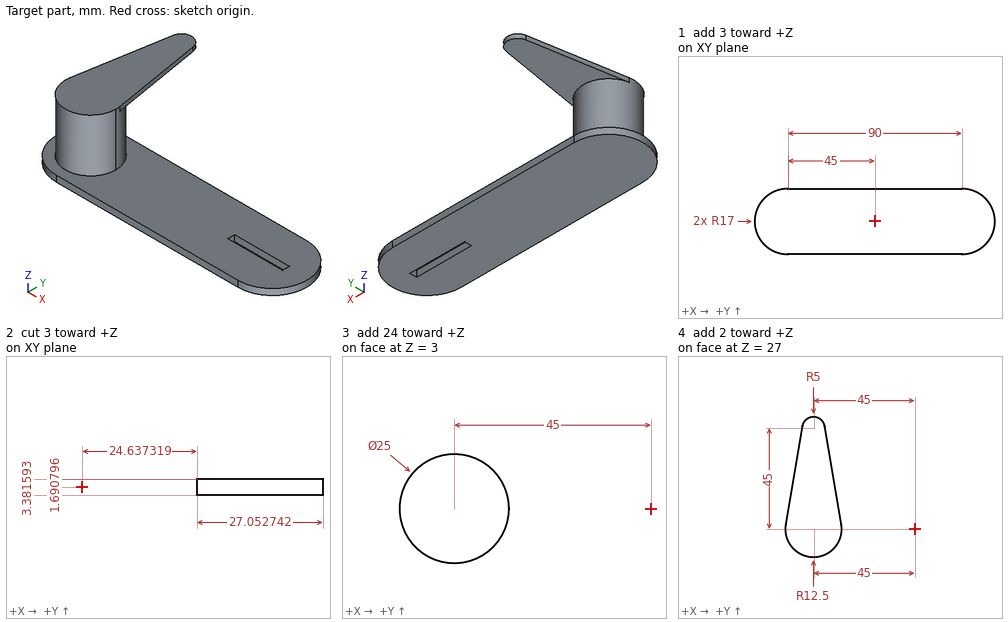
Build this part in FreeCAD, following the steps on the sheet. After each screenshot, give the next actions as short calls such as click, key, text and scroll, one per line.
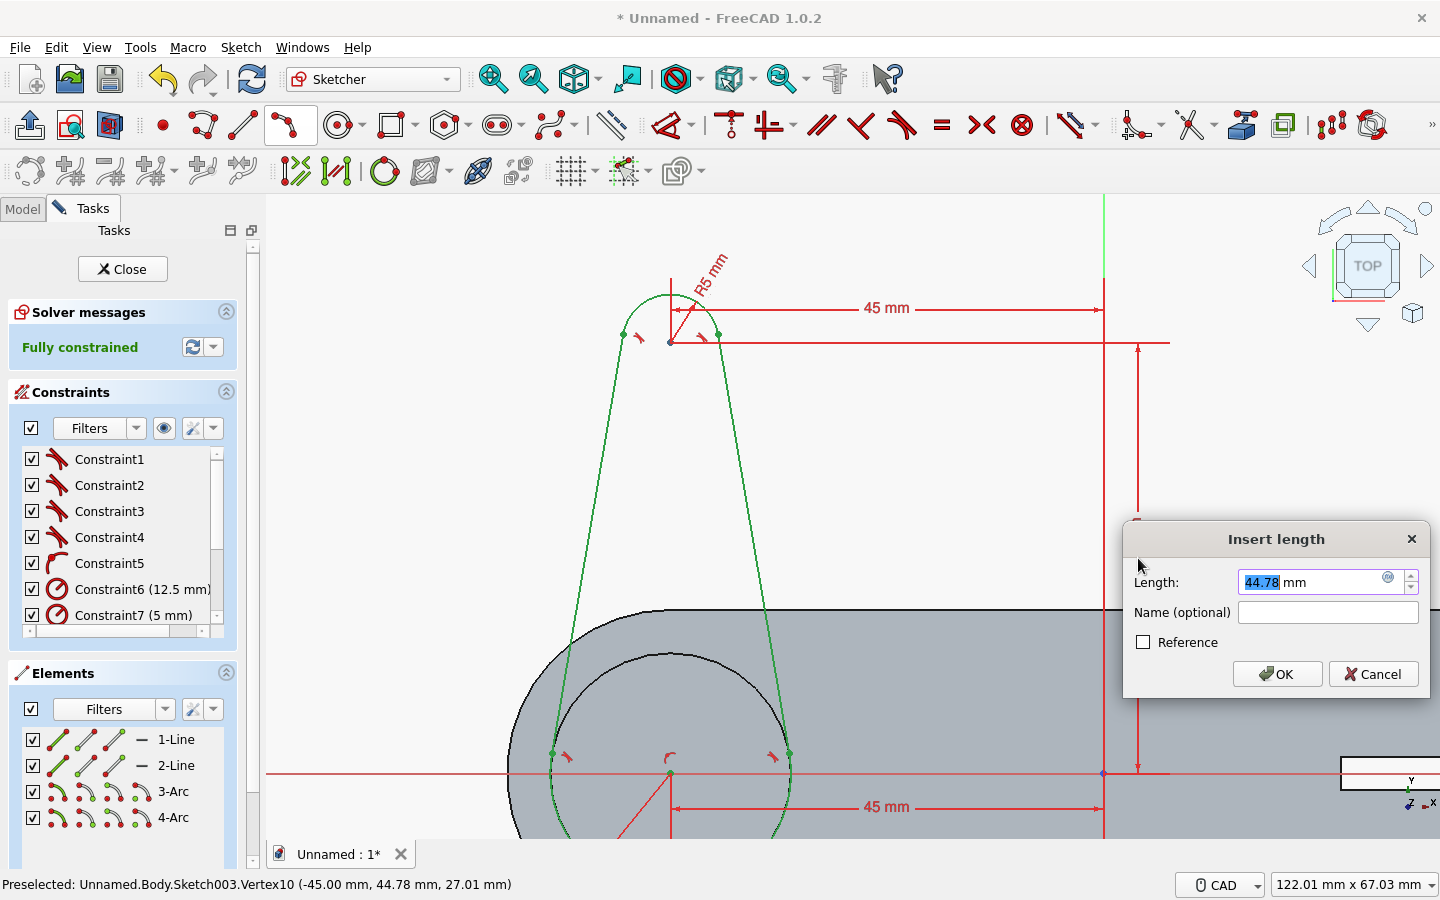
text(45)
key(Return)
key(Escape)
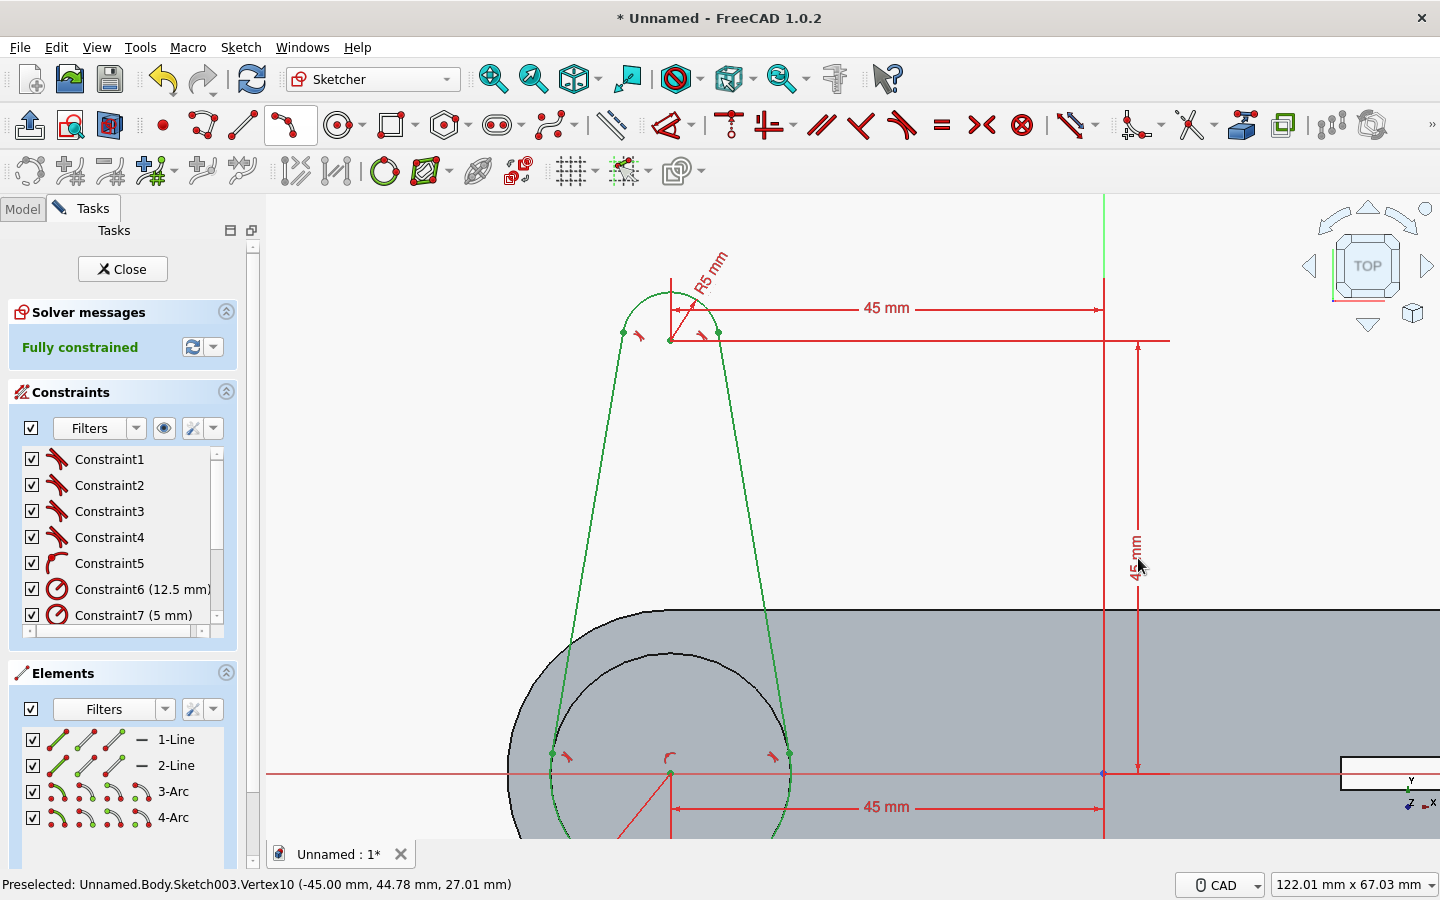
click(123, 269)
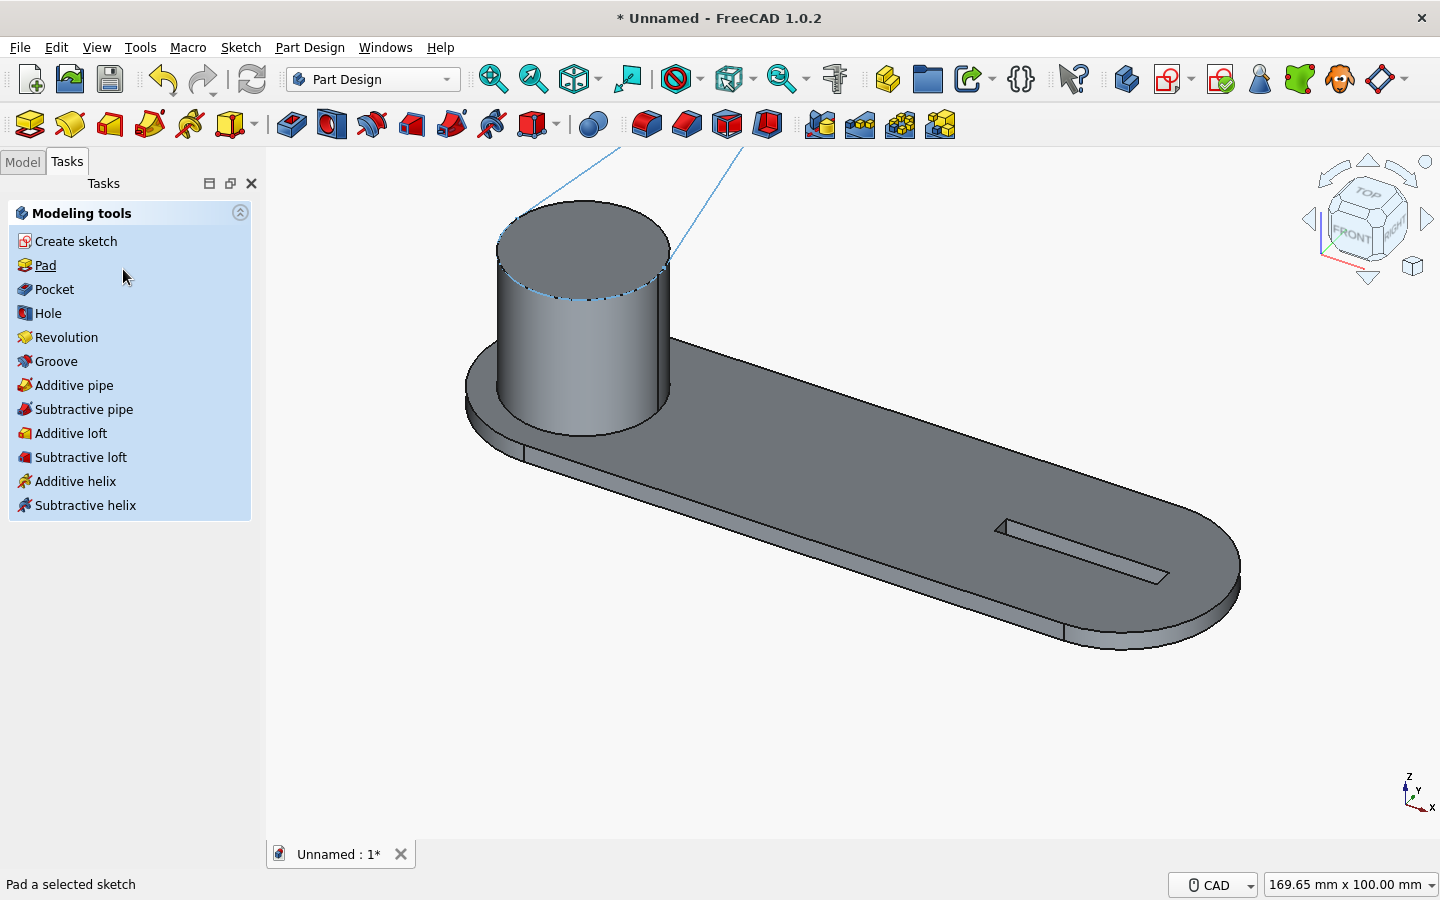
click(30, 124)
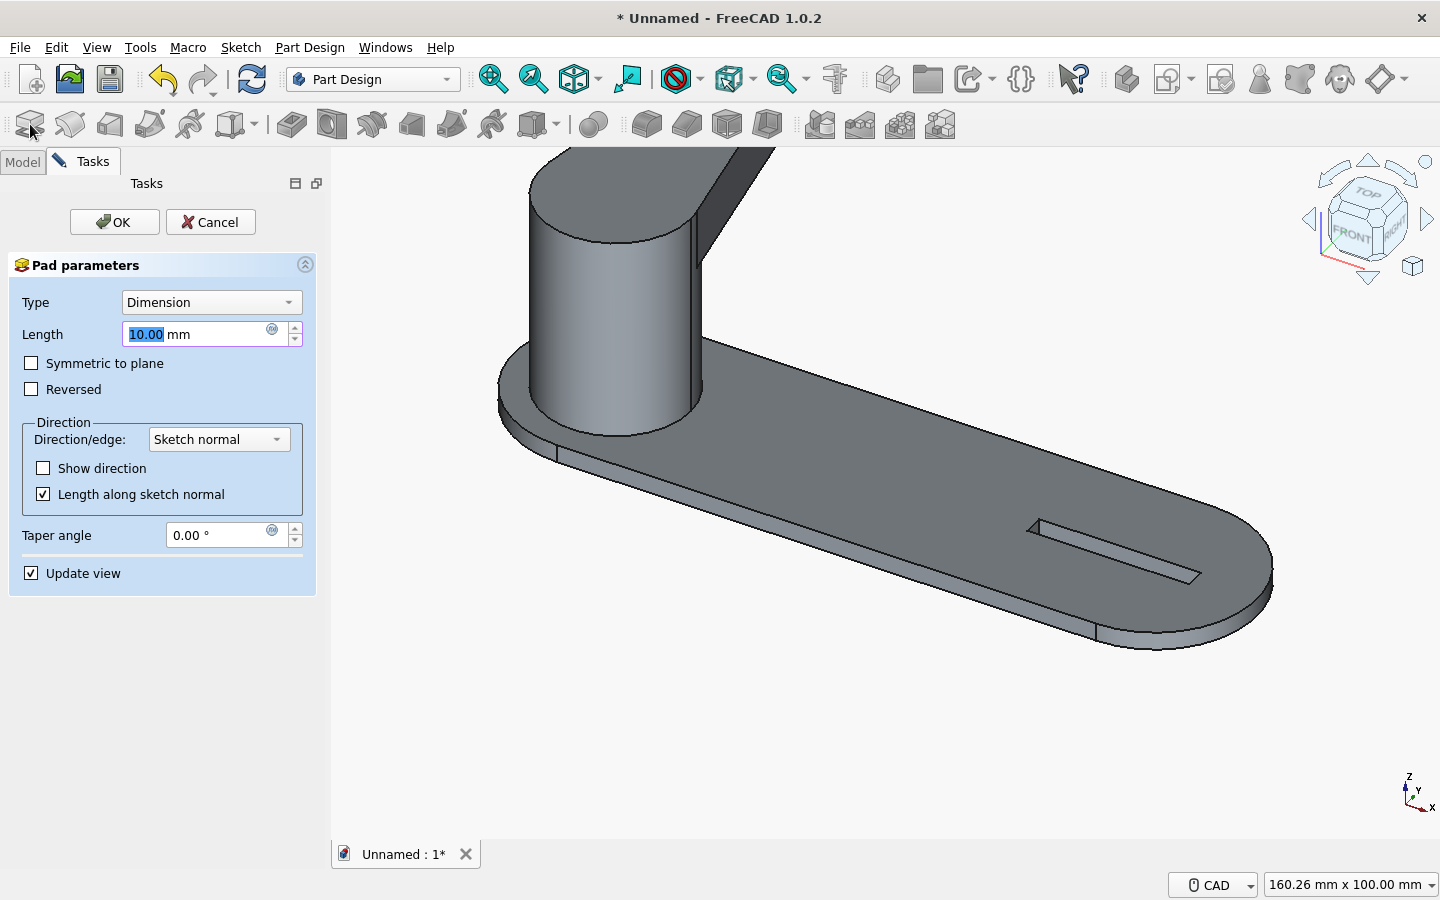
text(2)
key(Tab)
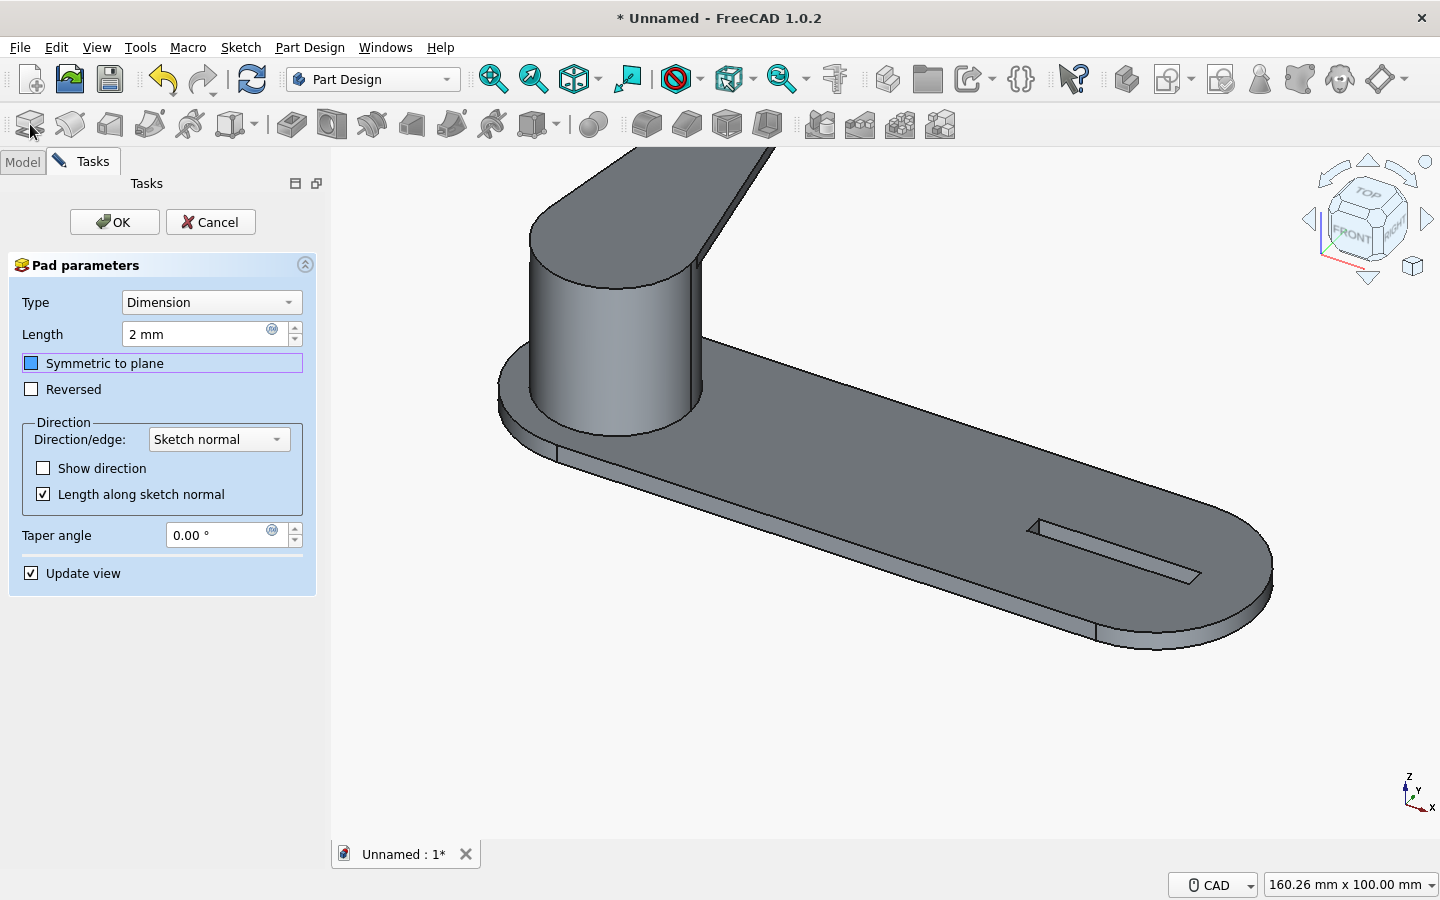
click(115, 222)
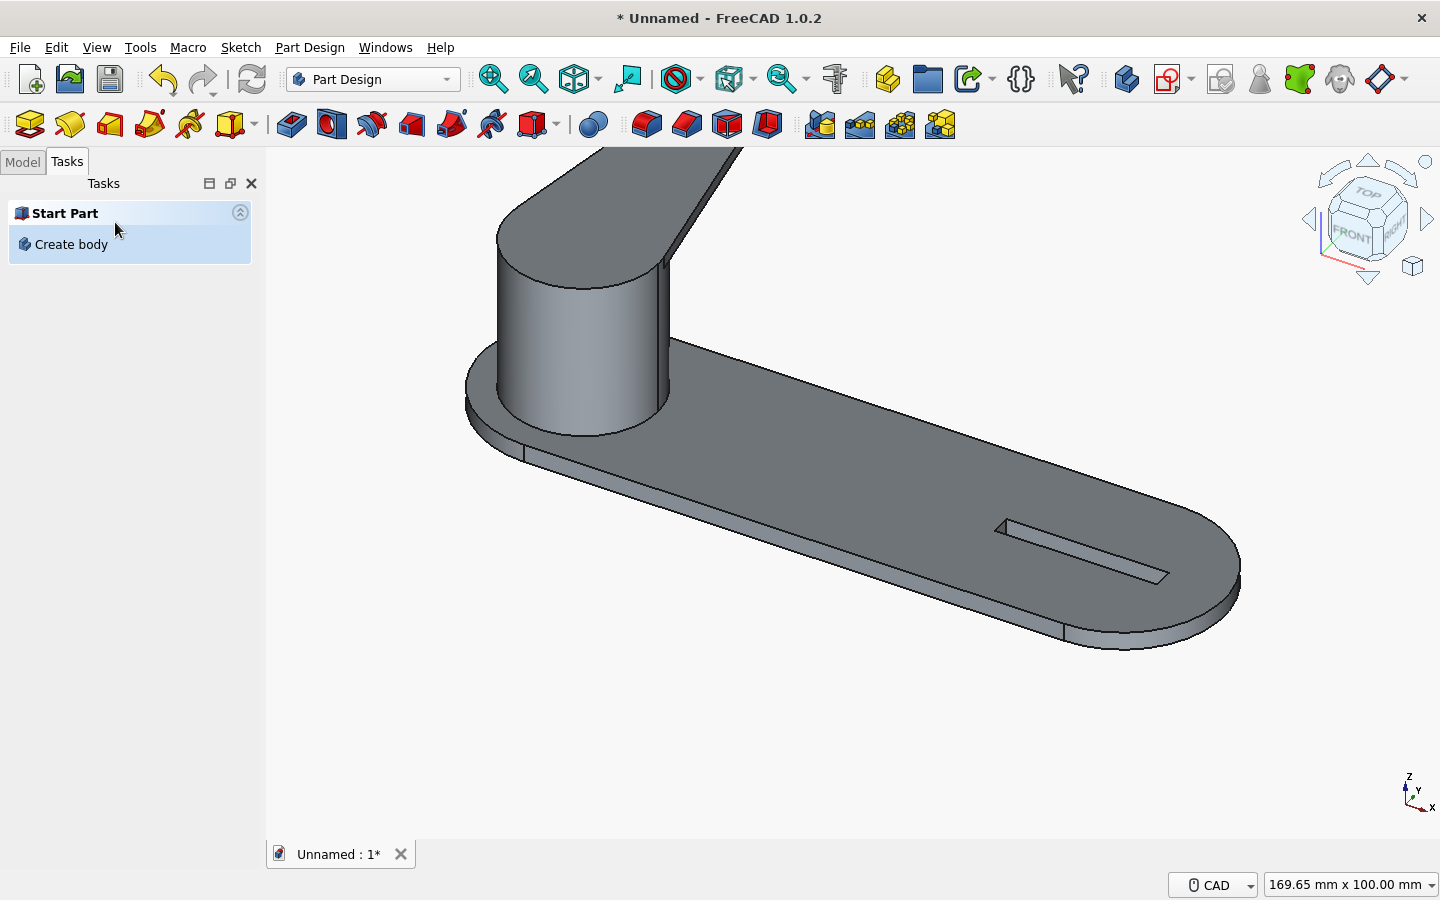
key(0)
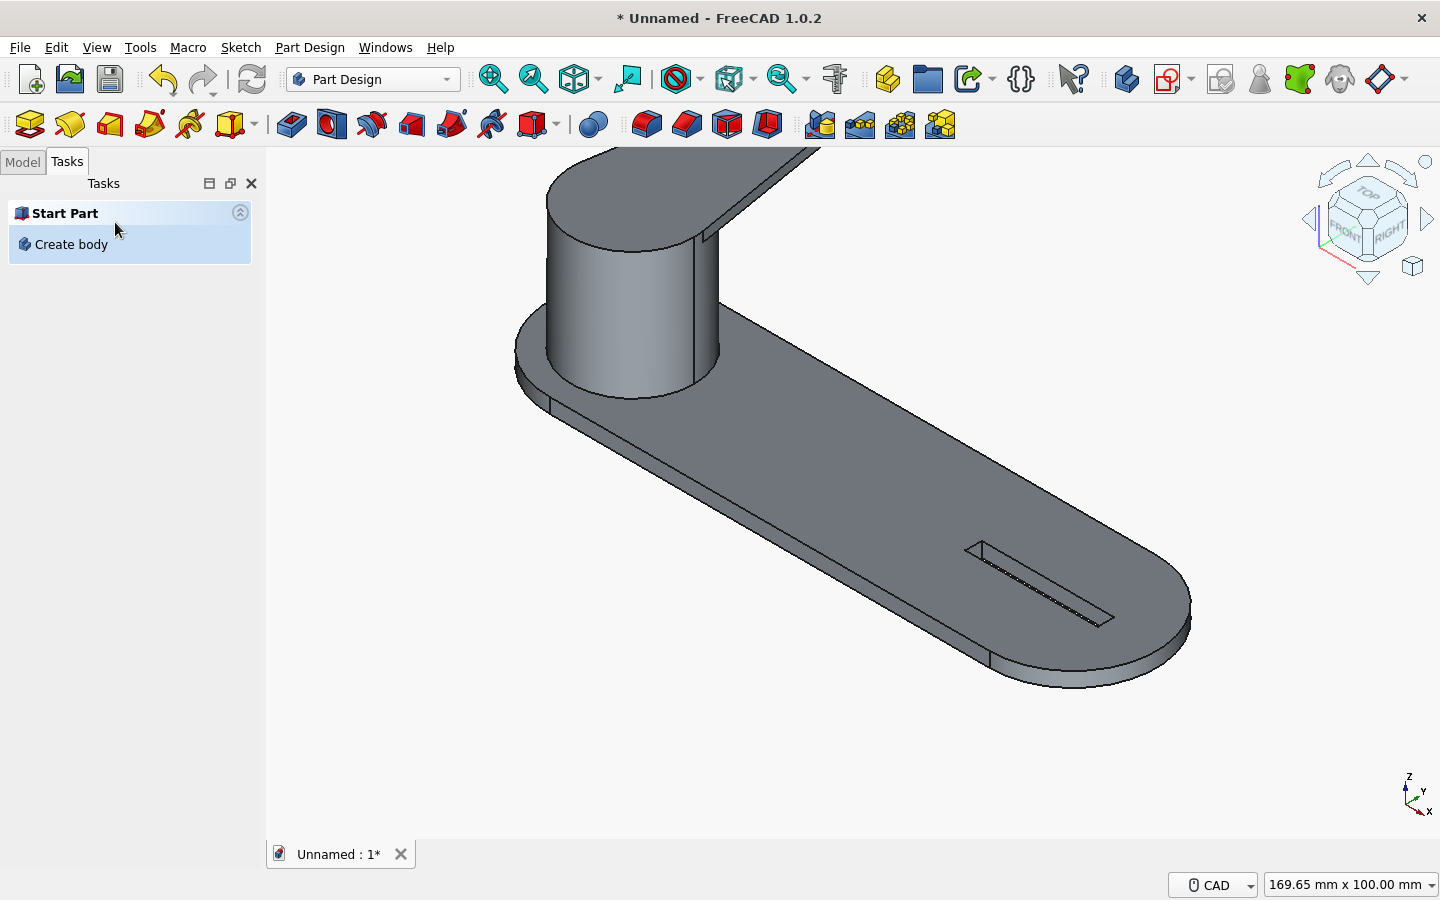
click(494, 80)